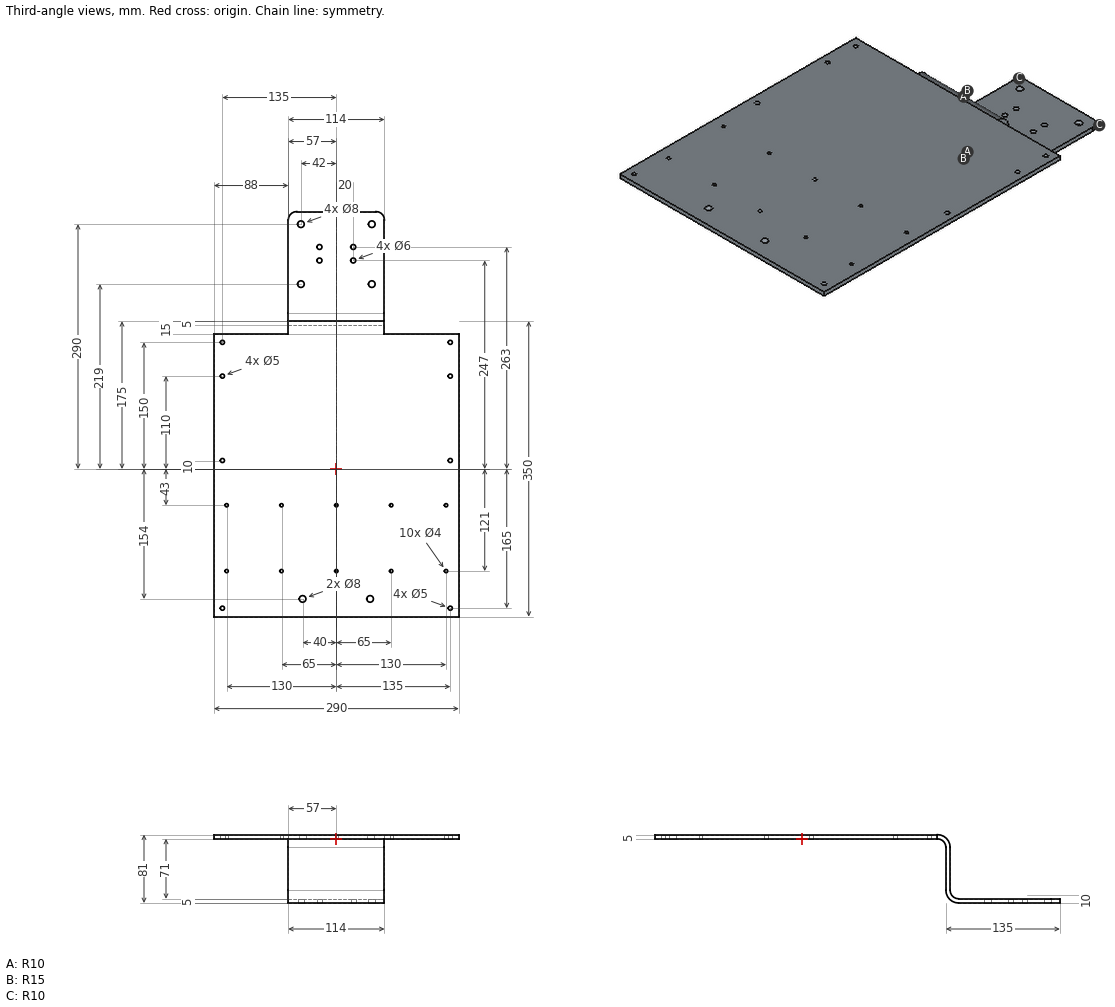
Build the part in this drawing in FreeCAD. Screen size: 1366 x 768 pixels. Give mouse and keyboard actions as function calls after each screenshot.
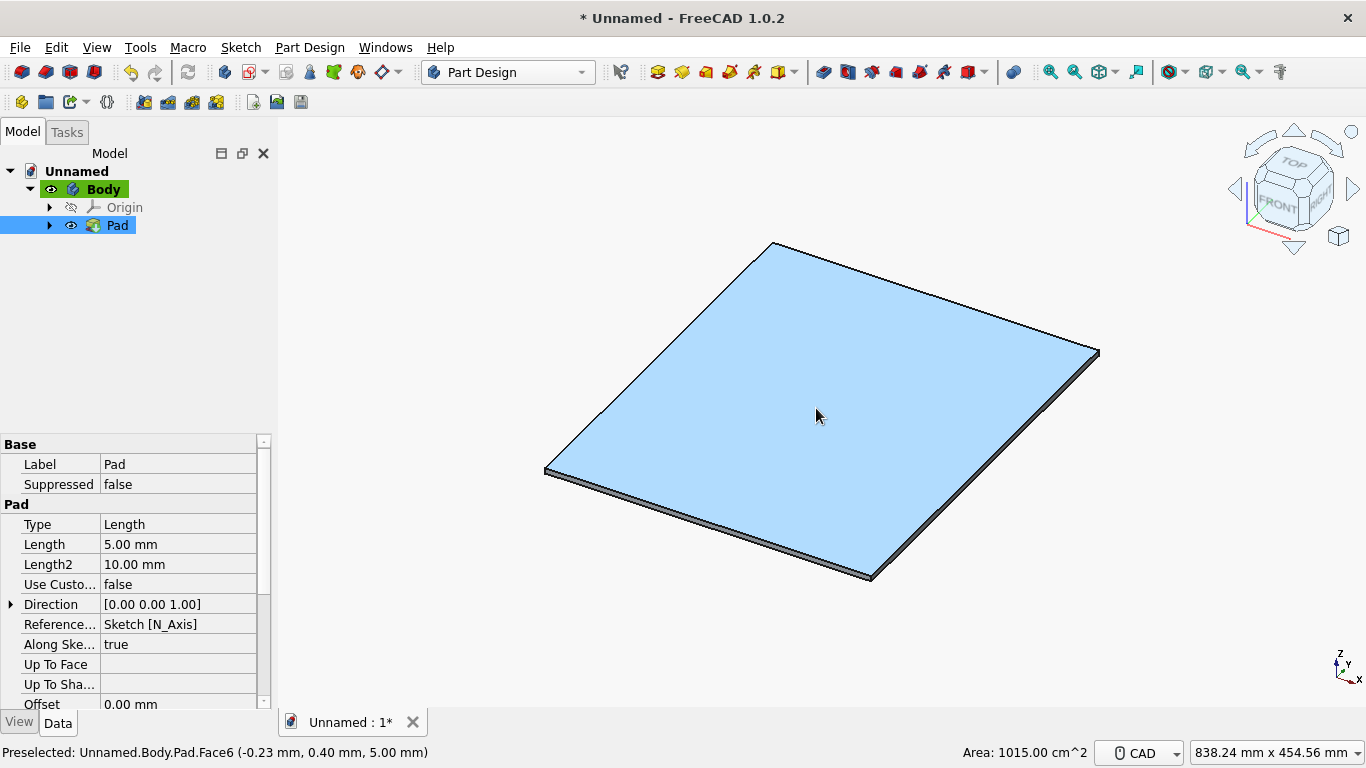
click(250, 72)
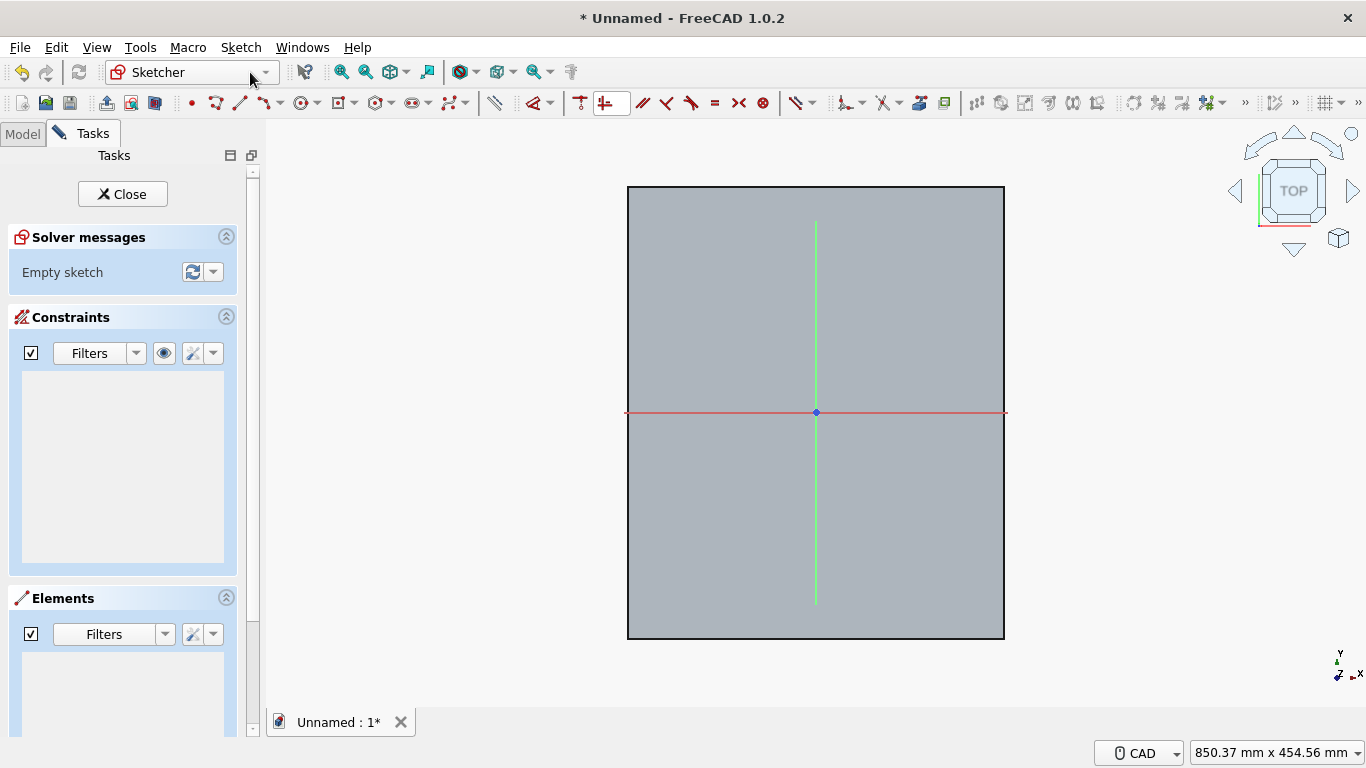
scroll(899, 162, up, 3)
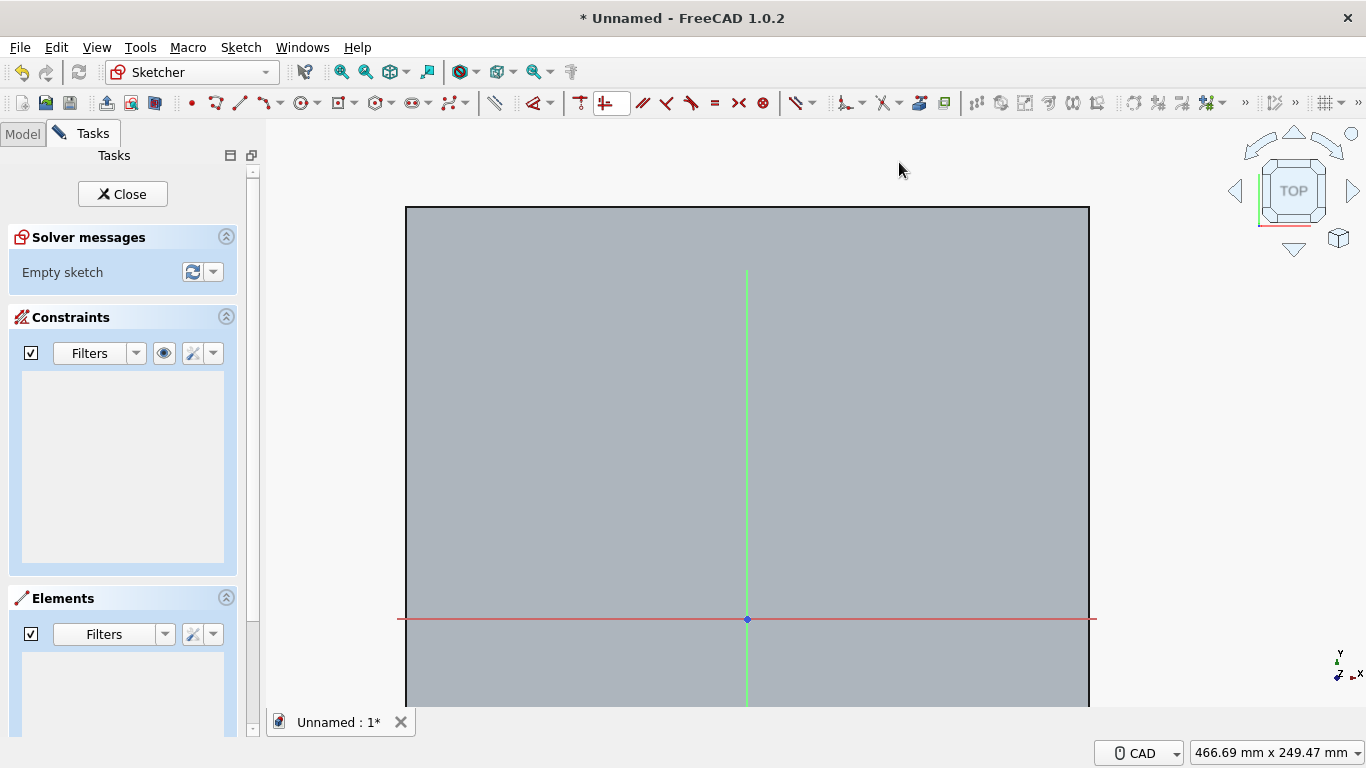
key(g)
key(r)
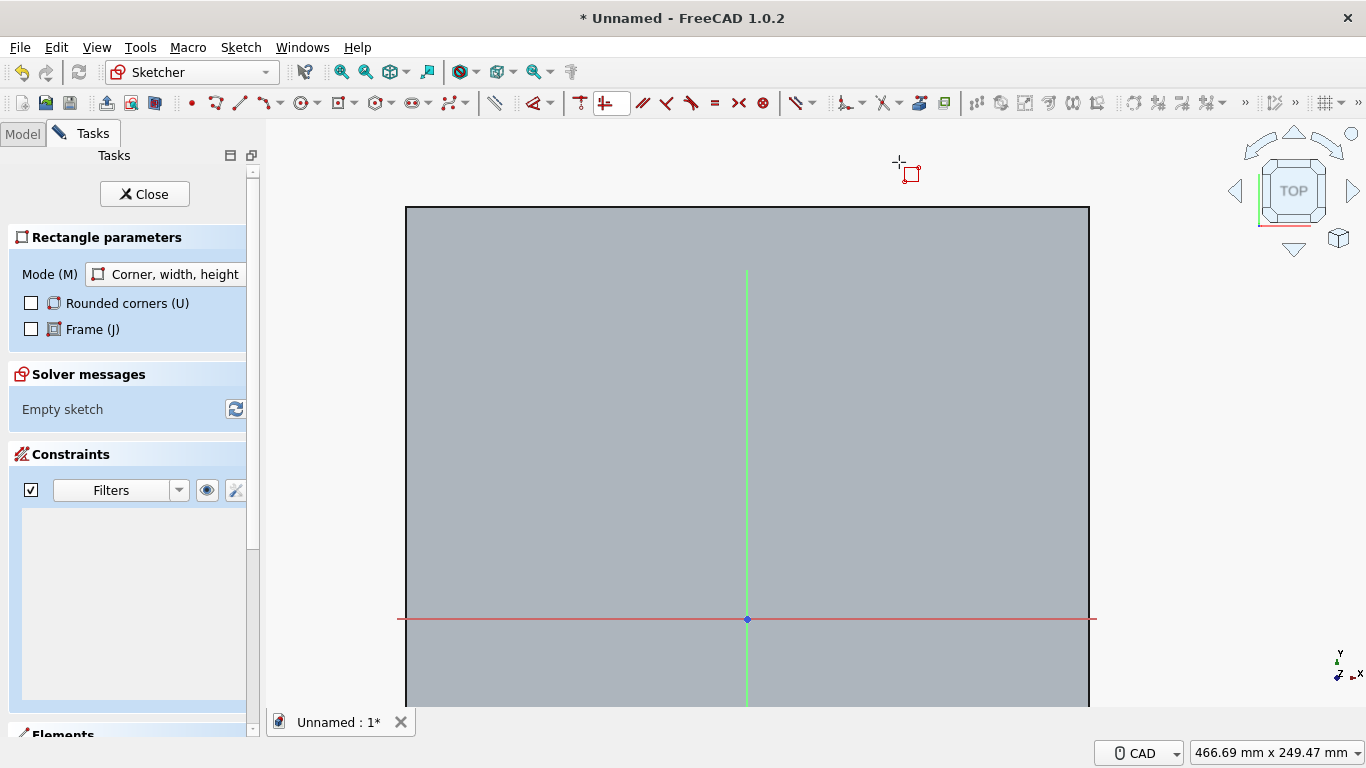
scroll(613, 207, up, 2)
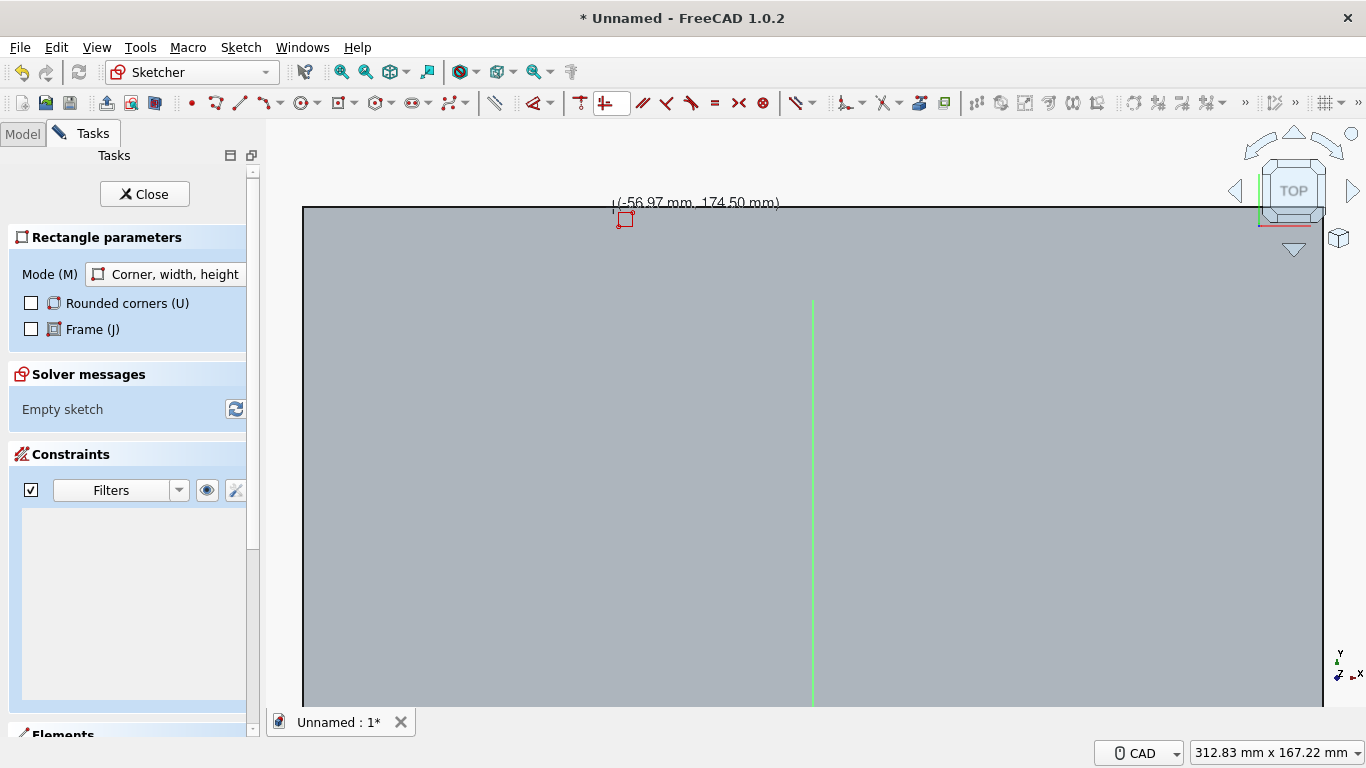
click(613, 207)
click(1014, 224)
key(Escape)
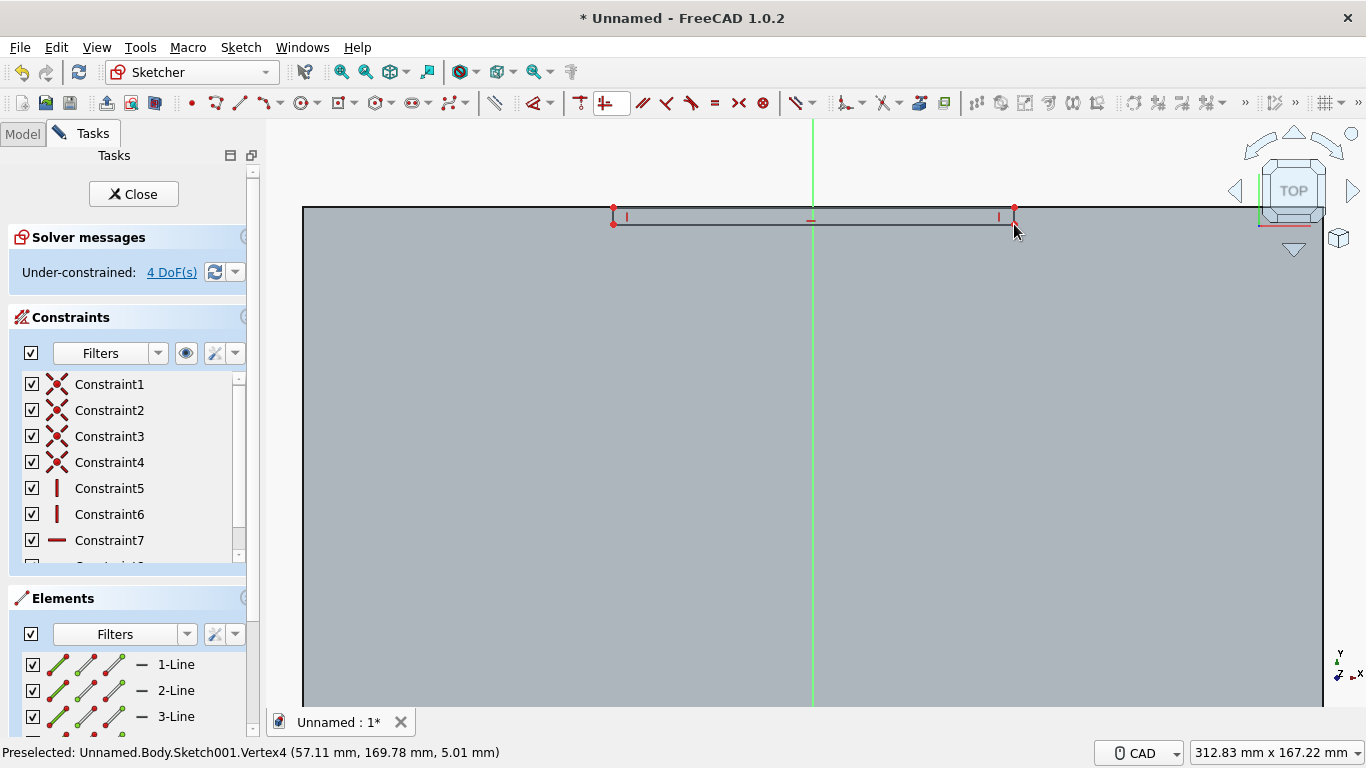
click(534, 104)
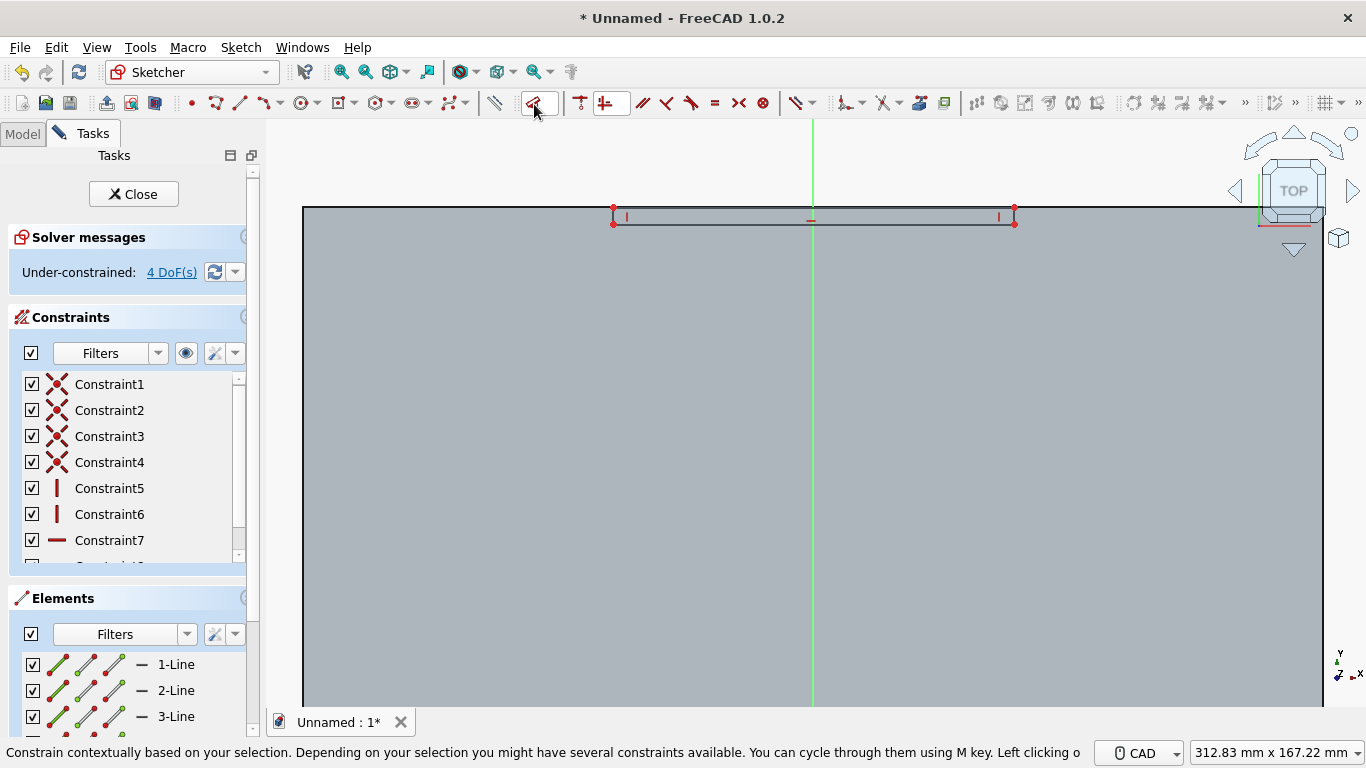
scroll(613, 217, up, 5)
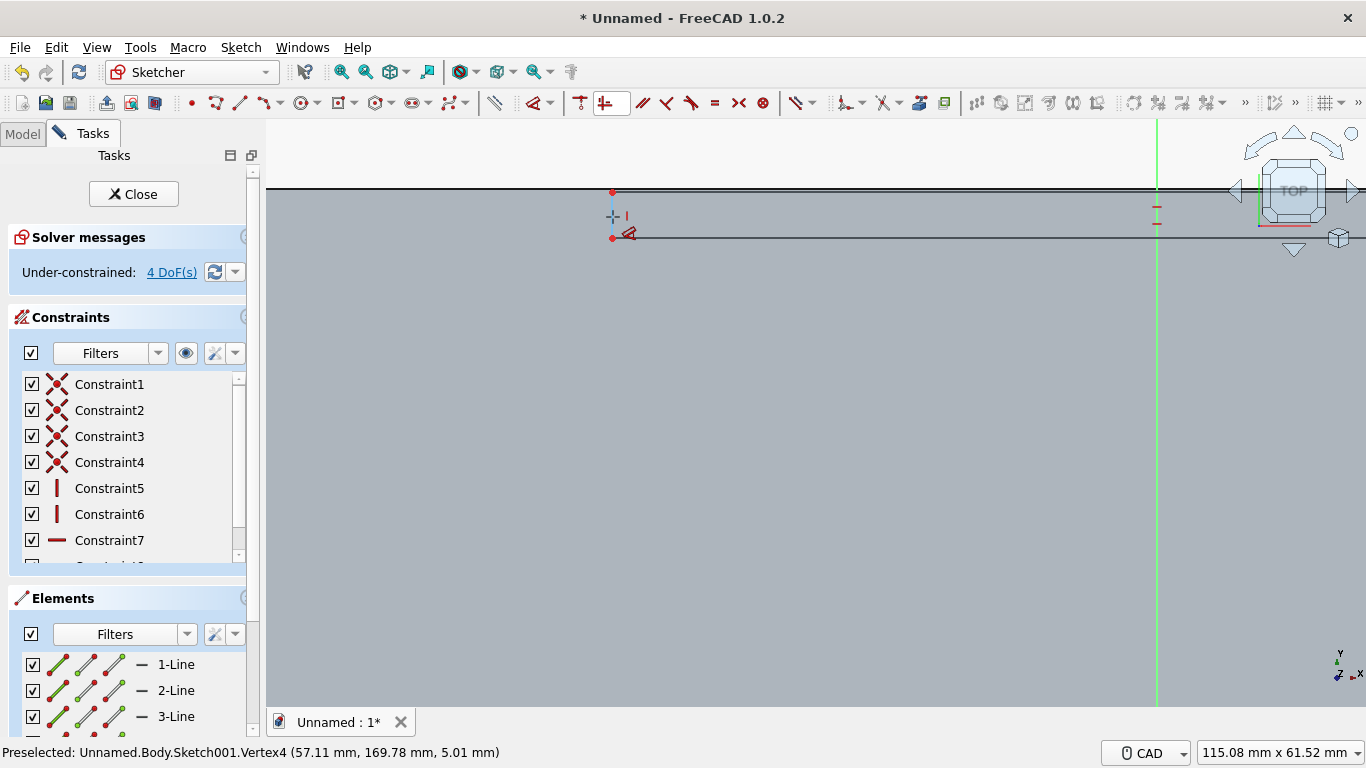
click(612, 215)
click(578, 215)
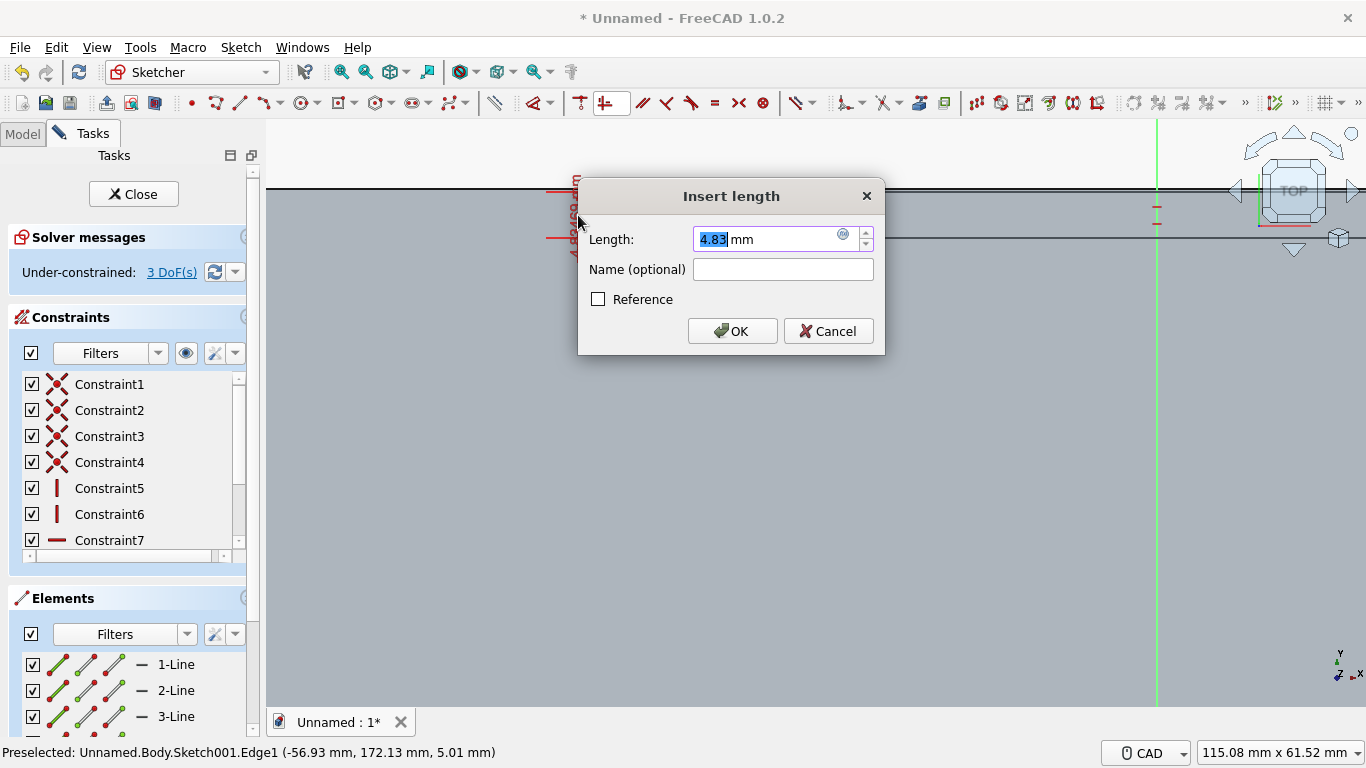
text(5)
key(Return)